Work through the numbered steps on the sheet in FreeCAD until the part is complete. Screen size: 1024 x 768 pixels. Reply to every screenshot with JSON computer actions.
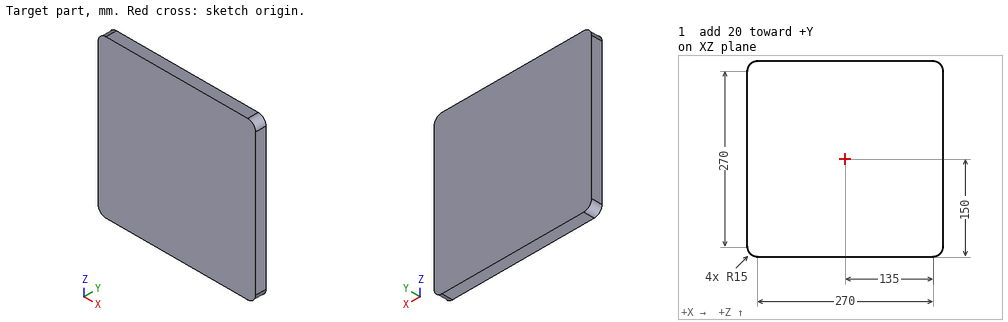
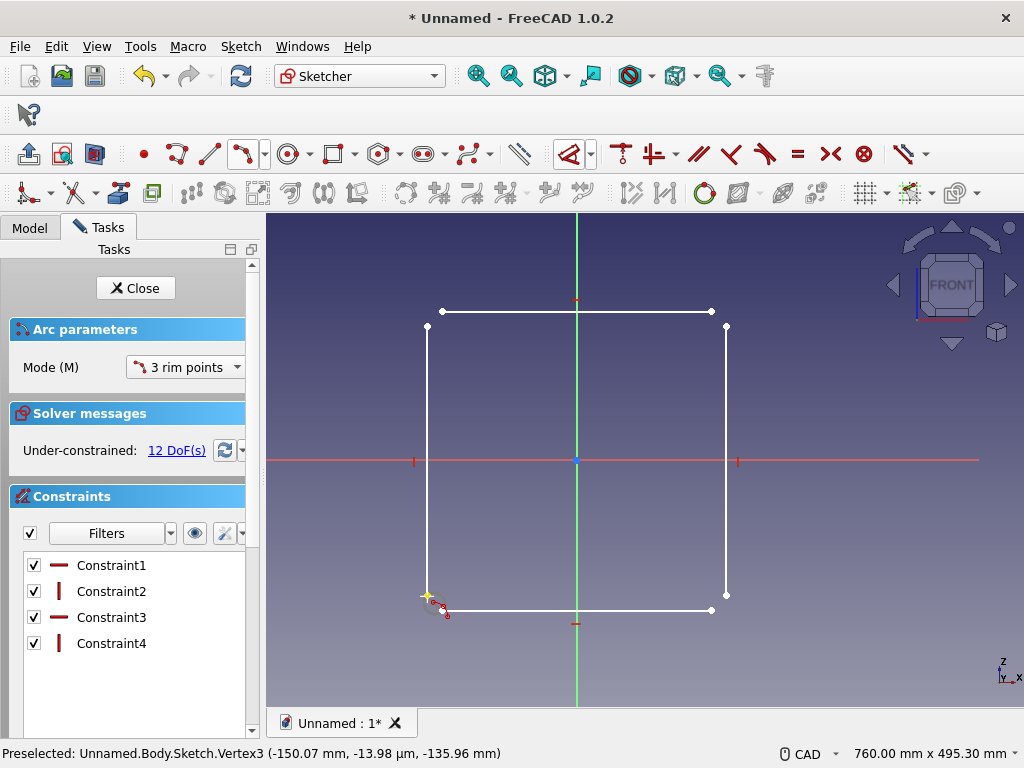
{"action": "scroll", "coordinate": [431, 606], "scroll_direction": "up", "scroll_amount": 7}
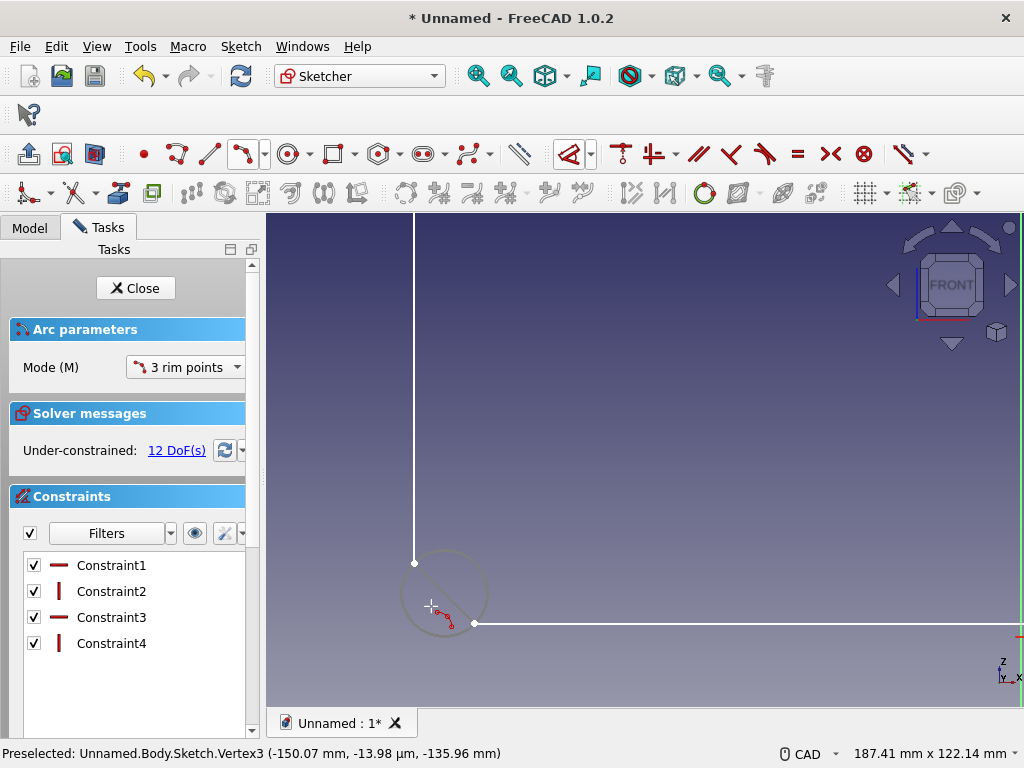
{"action": "left_click", "coordinate": [432, 602]}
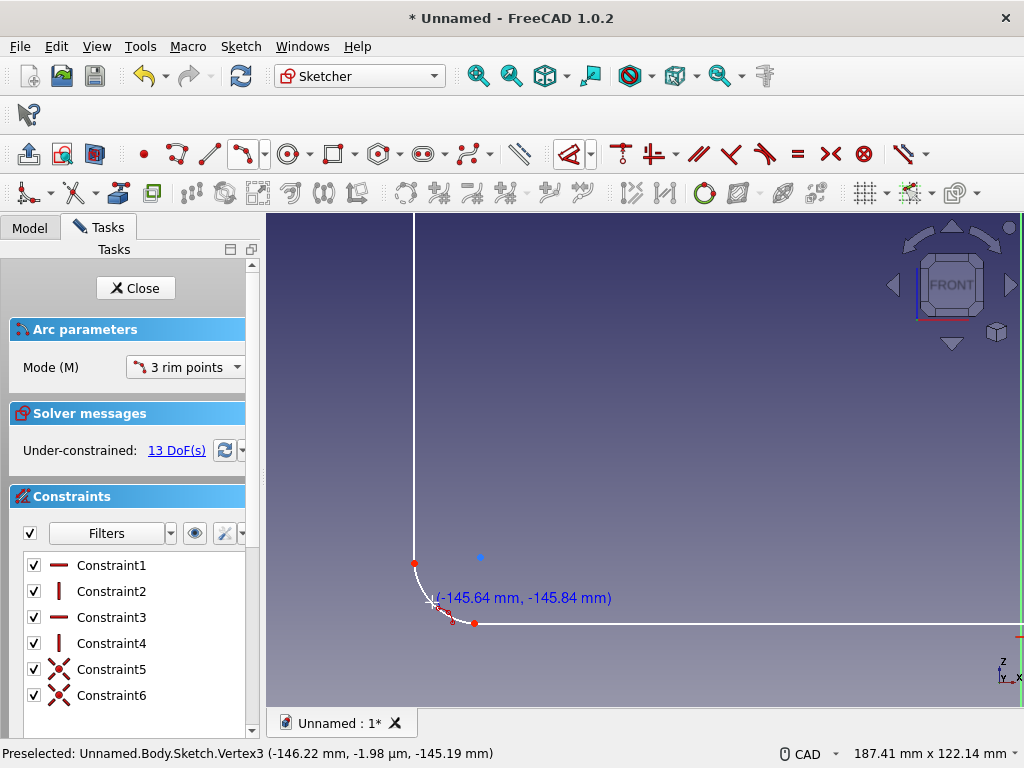
{"action": "scroll", "coordinate": [431, 606], "scroll_direction": "down", "scroll_amount": 7}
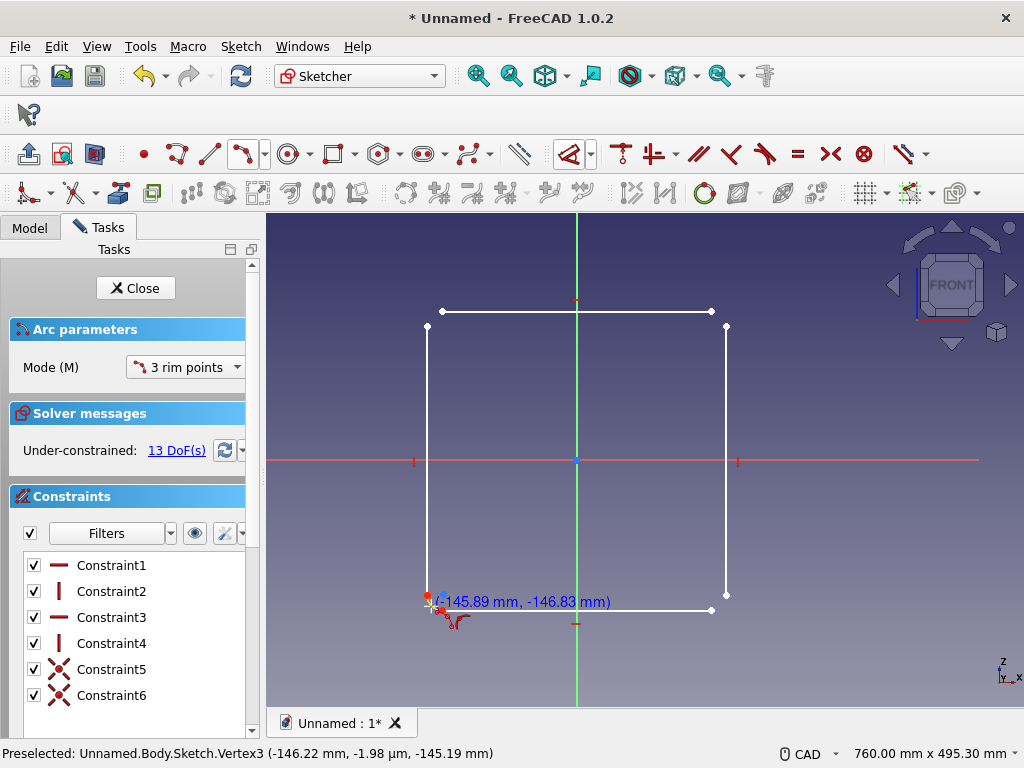
{"action": "left_click", "coordinate": [427, 327]}
{"action": "left_click", "coordinate": [442, 312]}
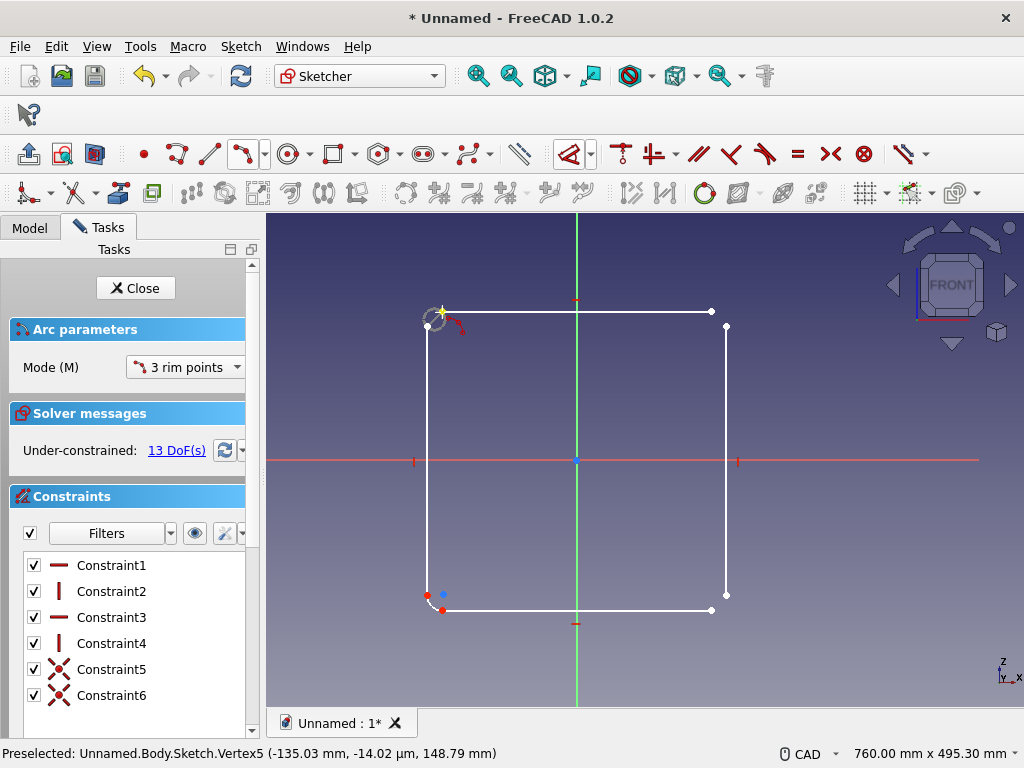
{"action": "scroll", "coordinate": [431, 315], "scroll_direction": "up", "scroll_amount": 7}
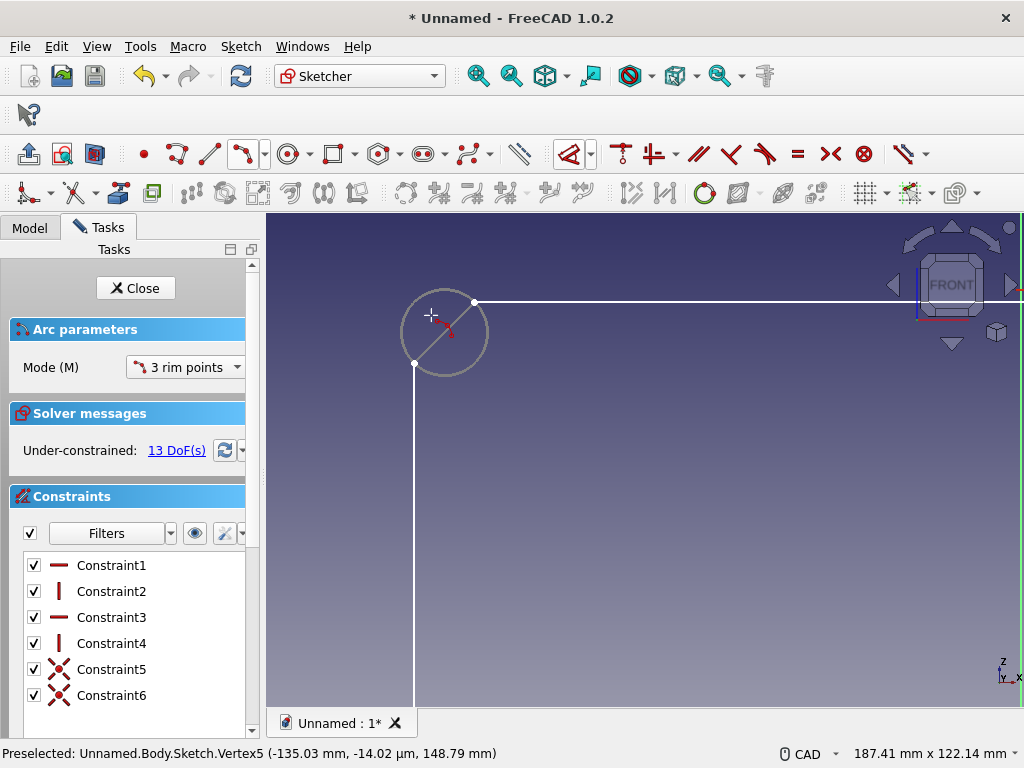
{"action": "left_click", "coordinate": [432, 315]}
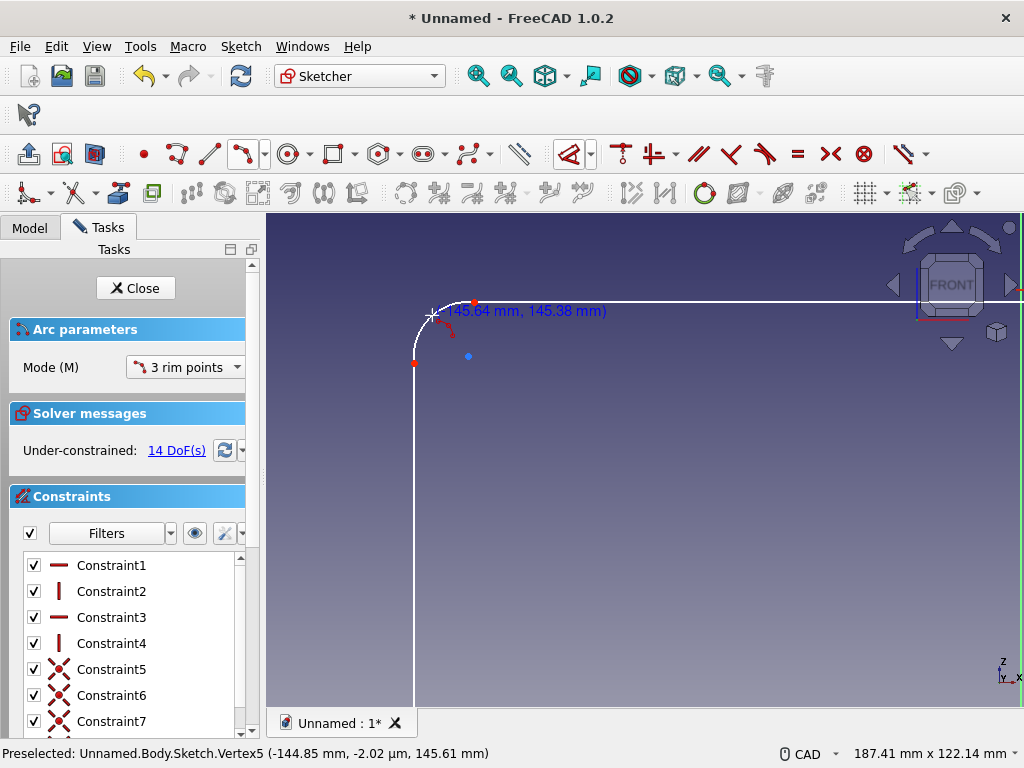
{"action": "scroll", "coordinate": [431, 315], "scroll_direction": "down", "scroll_amount": 7}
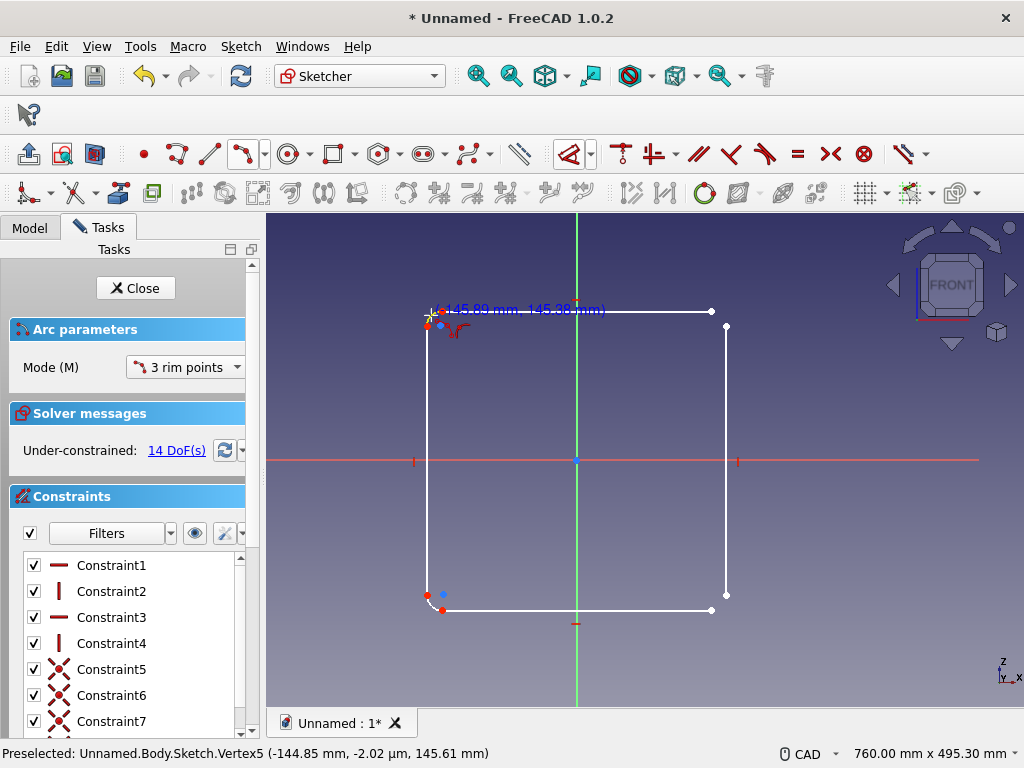
{"action": "left_click", "coordinate": [711, 312]}
{"action": "left_click", "coordinate": [726, 327]}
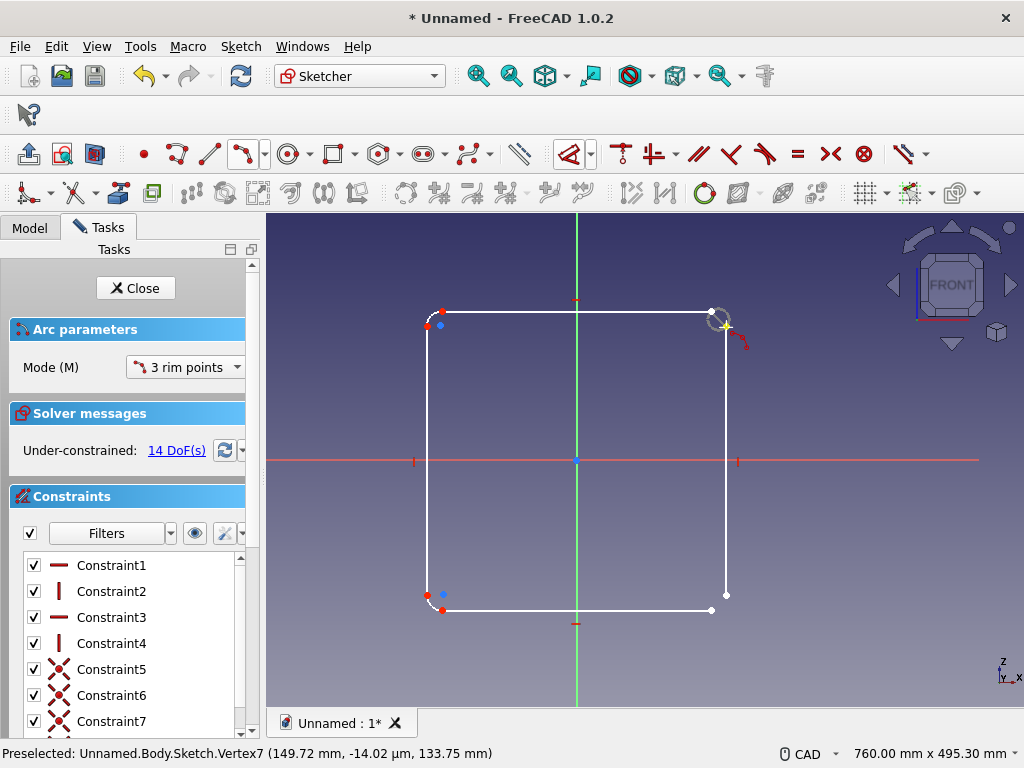
{"action": "scroll", "coordinate": [722, 315], "scroll_direction": "up", "scroll_amount": 7}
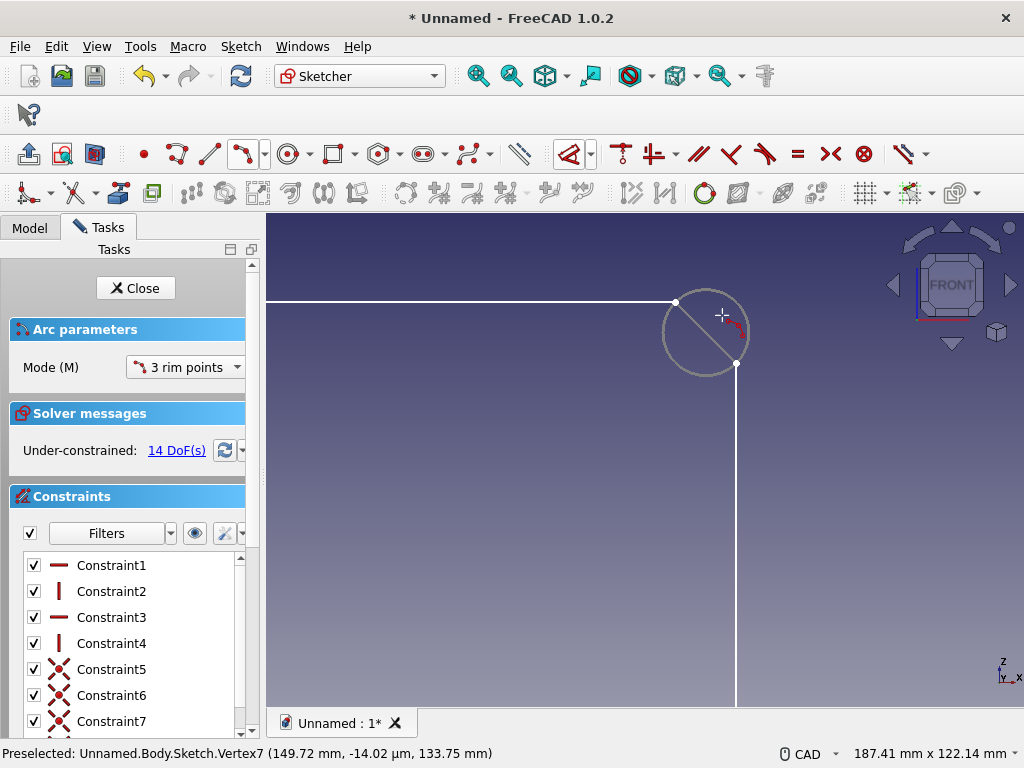
{"action": "left_click", "coordinate": [720, 315]}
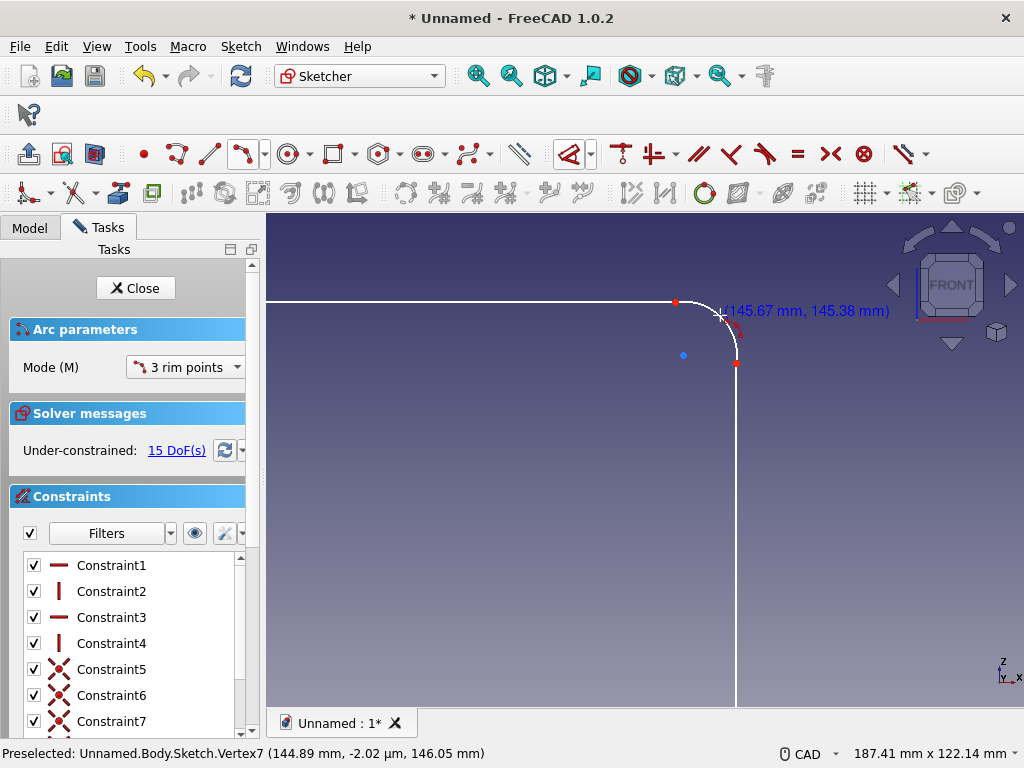
{"action": "scroll", "coordinate": [722, 315], "scroll_direction": "down", "scroll_amount": 7}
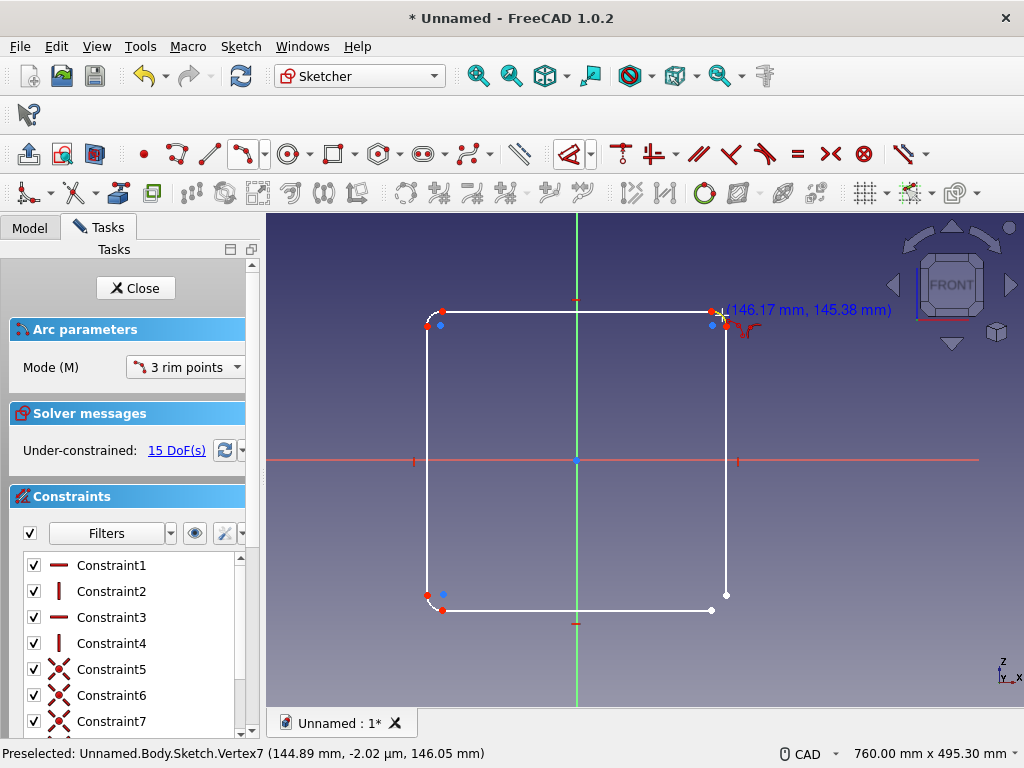
{"action": "left_click", "coordinate": [726, 596]}
{"action": "left_click", "coordinate": [711, 611]}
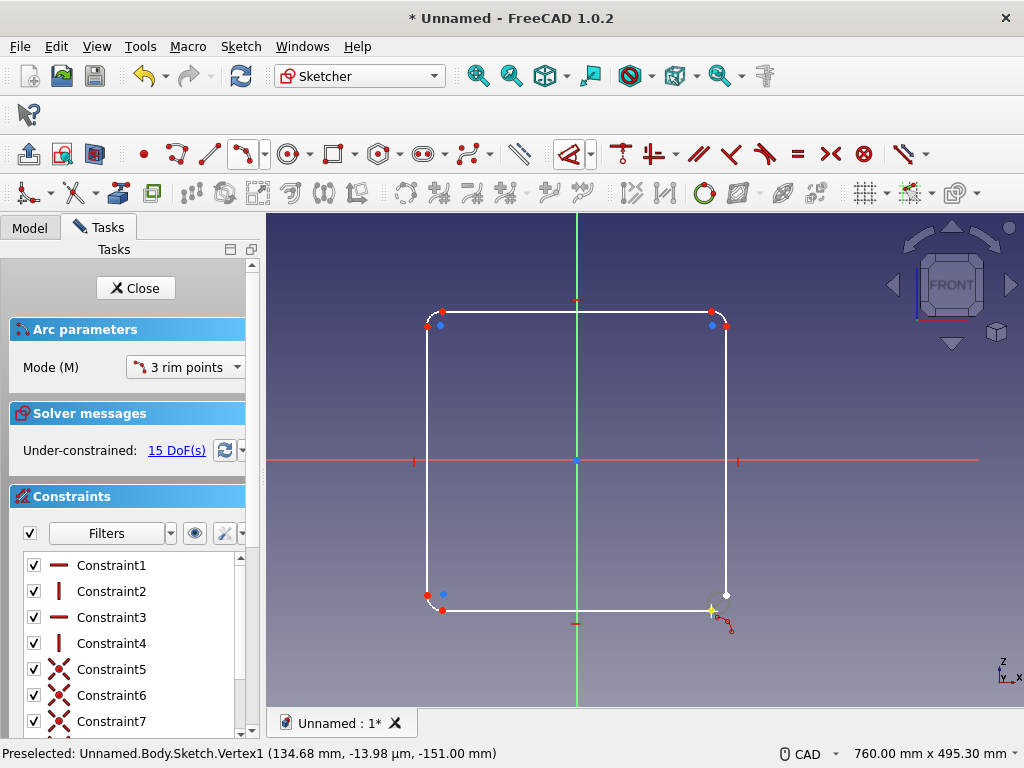
{"action": "scroll", "coordinate": [722, 606], "scroll_direction": "up", "scroll_amount": 7}